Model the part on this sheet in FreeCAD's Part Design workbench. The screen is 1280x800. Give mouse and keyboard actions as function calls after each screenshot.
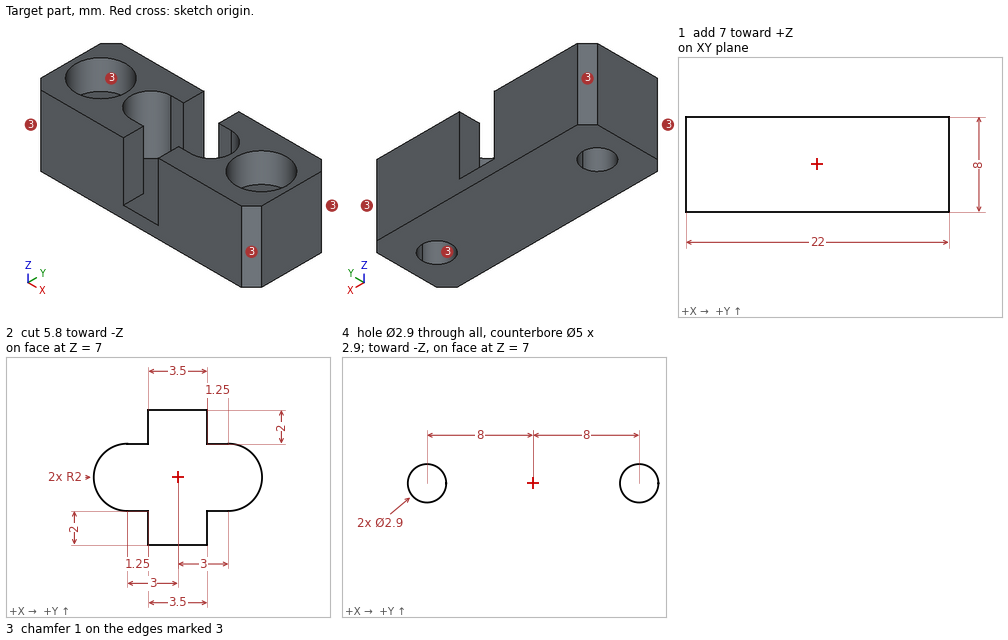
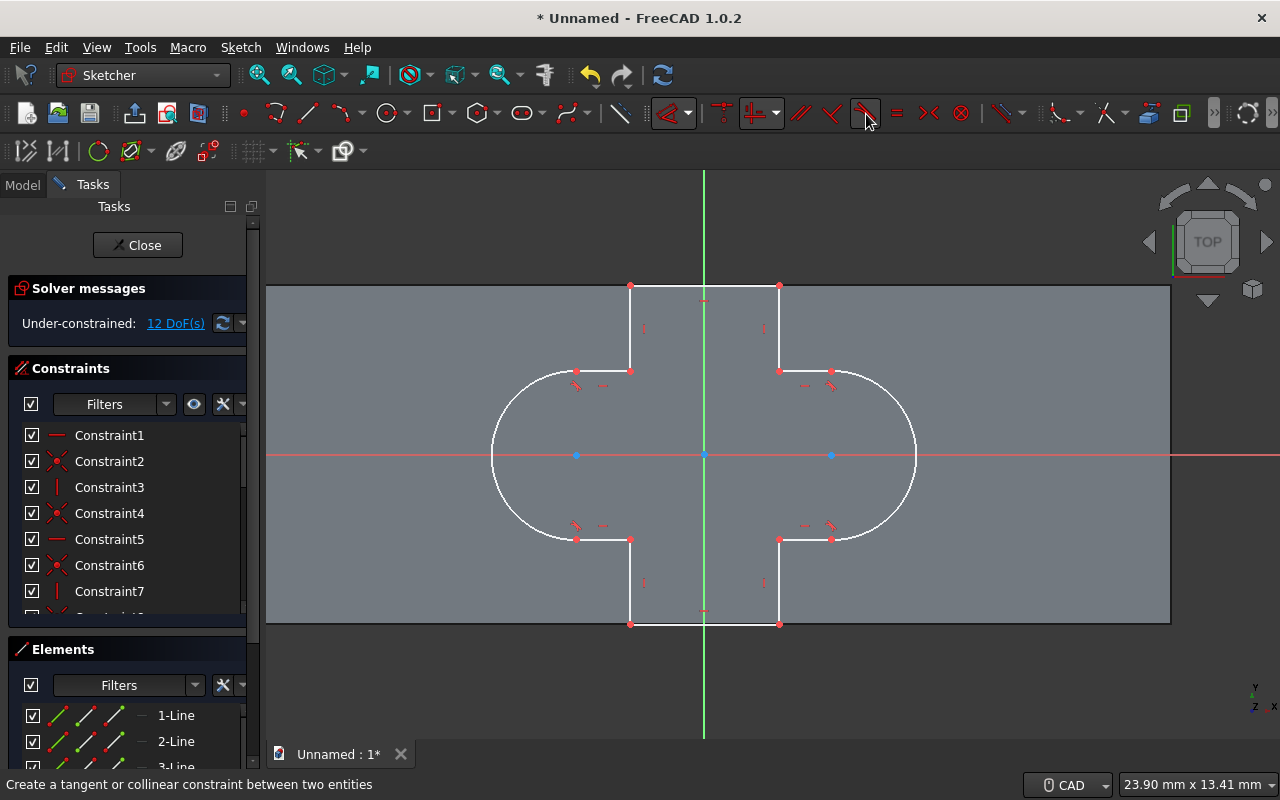
click(900, 505)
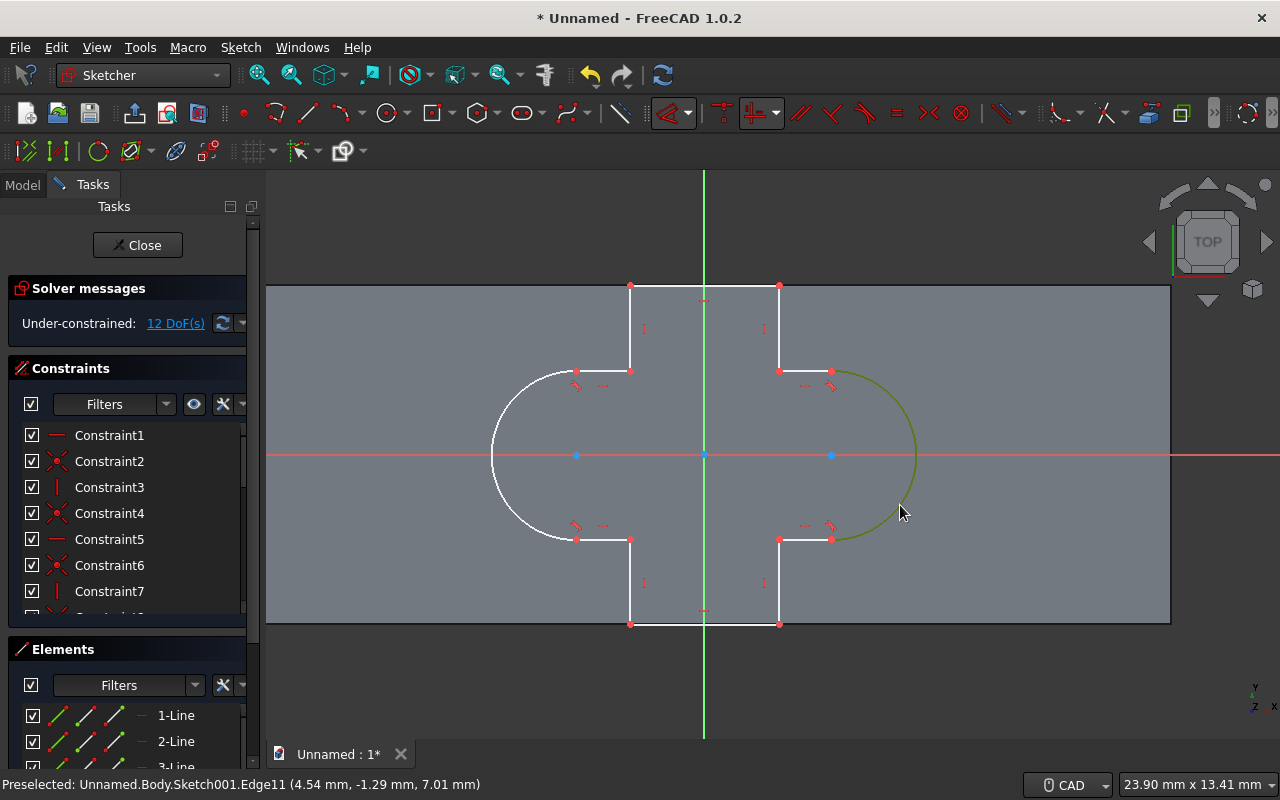
click(508, 406)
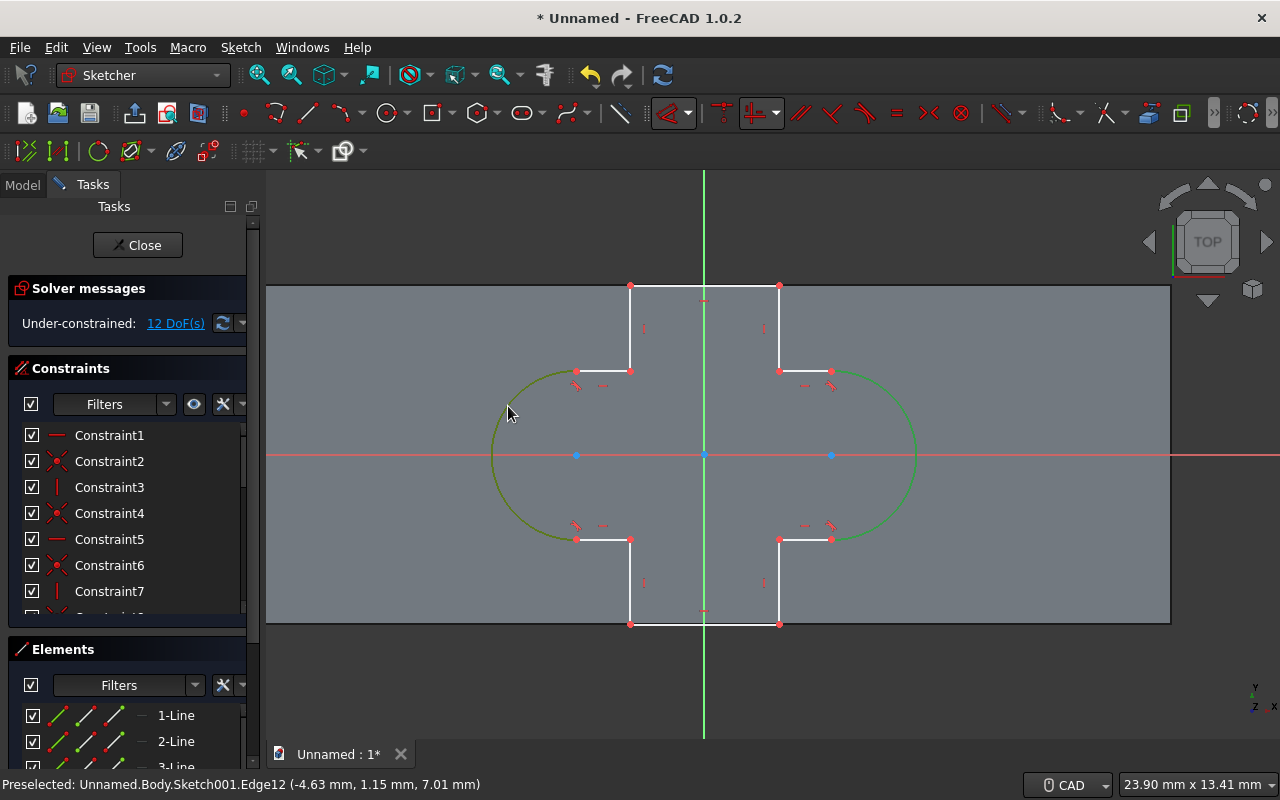
click(898, 114)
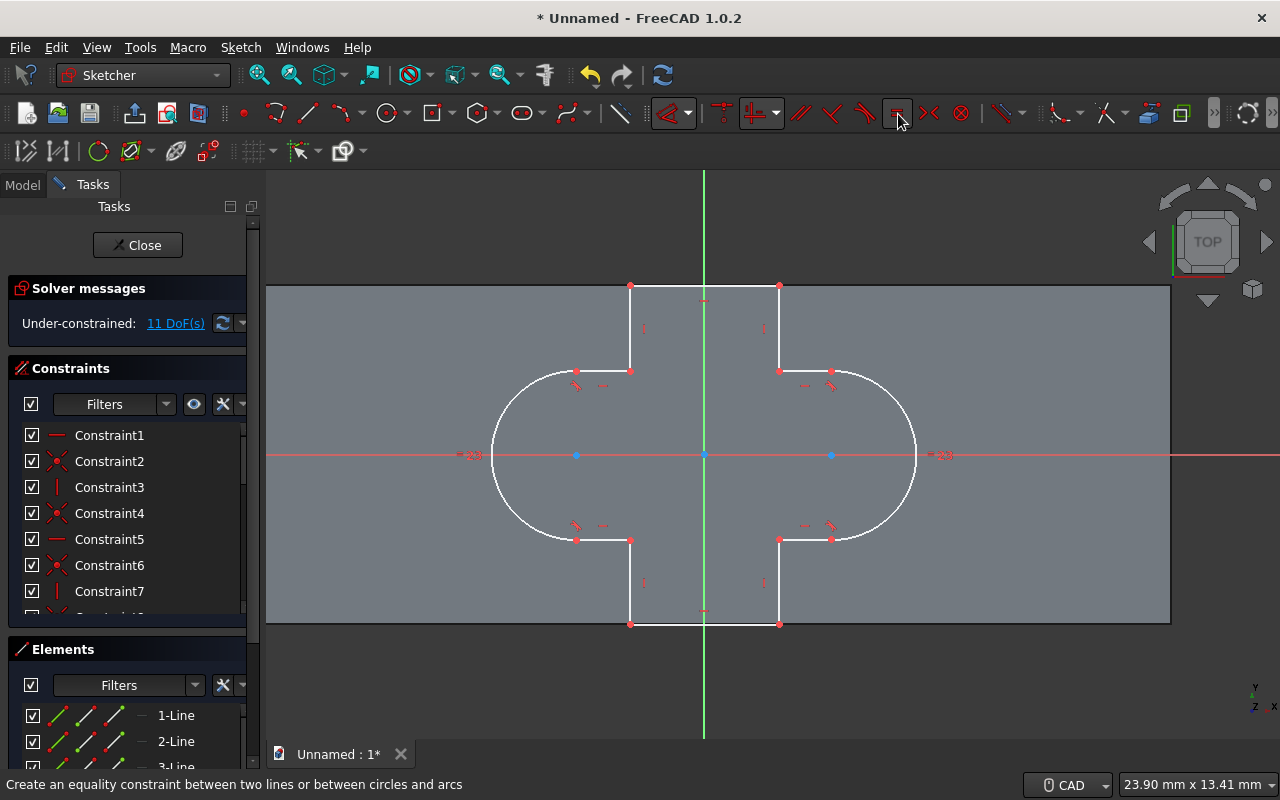
click(832, 456)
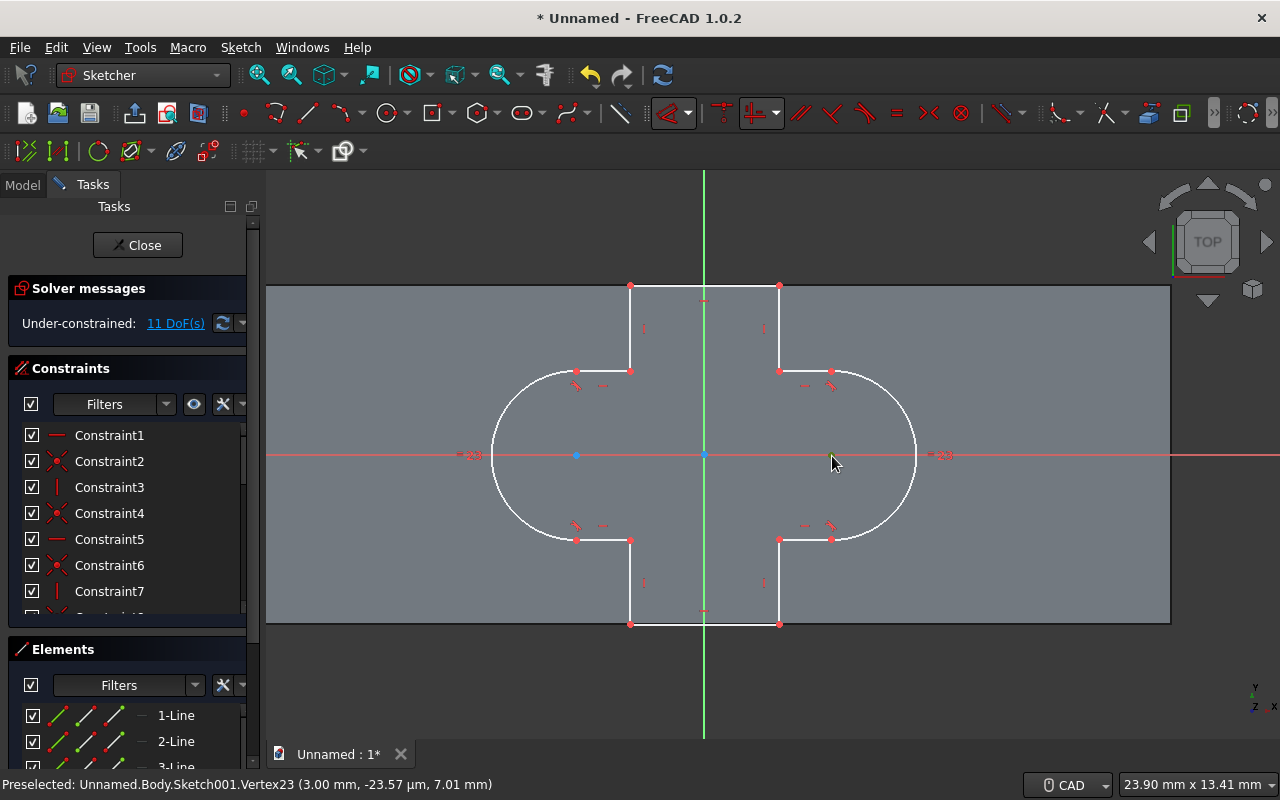
click(353, 454)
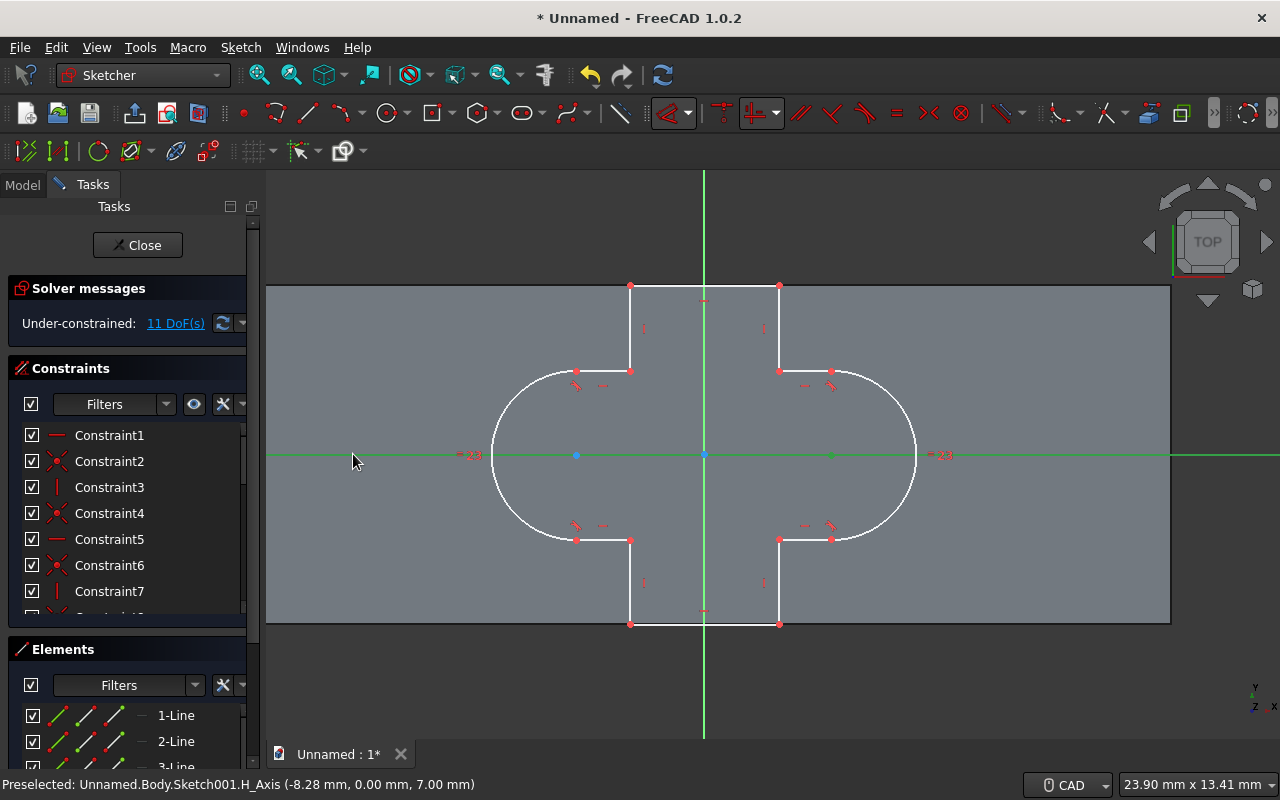
click(722, 114)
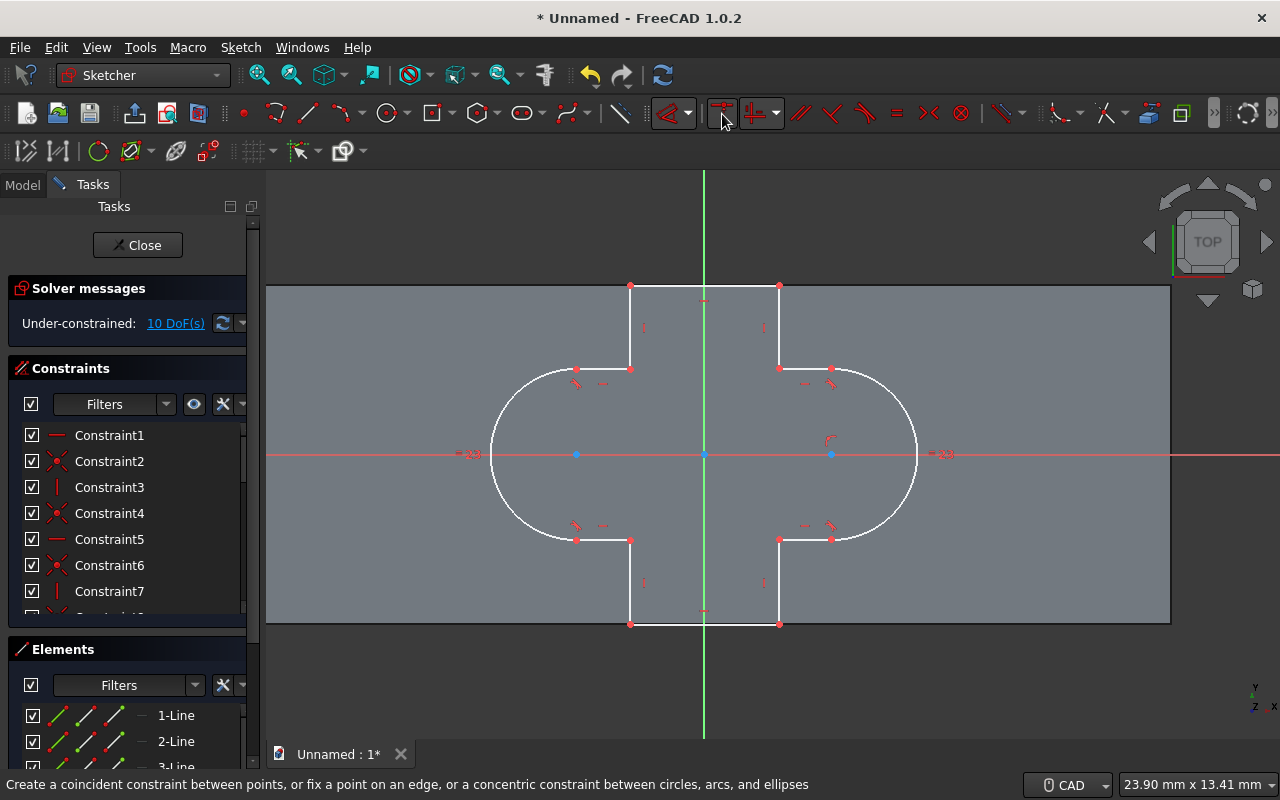
click(576, 455)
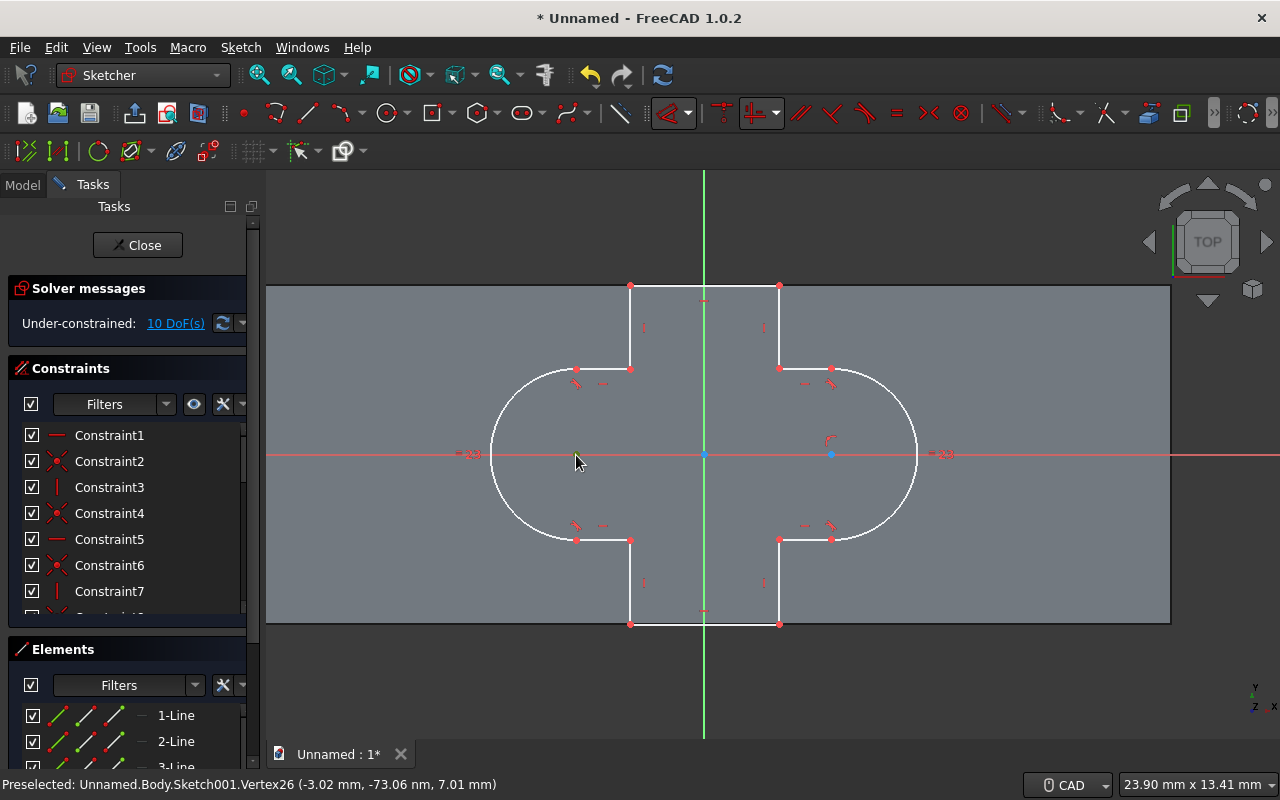
click(353, 454)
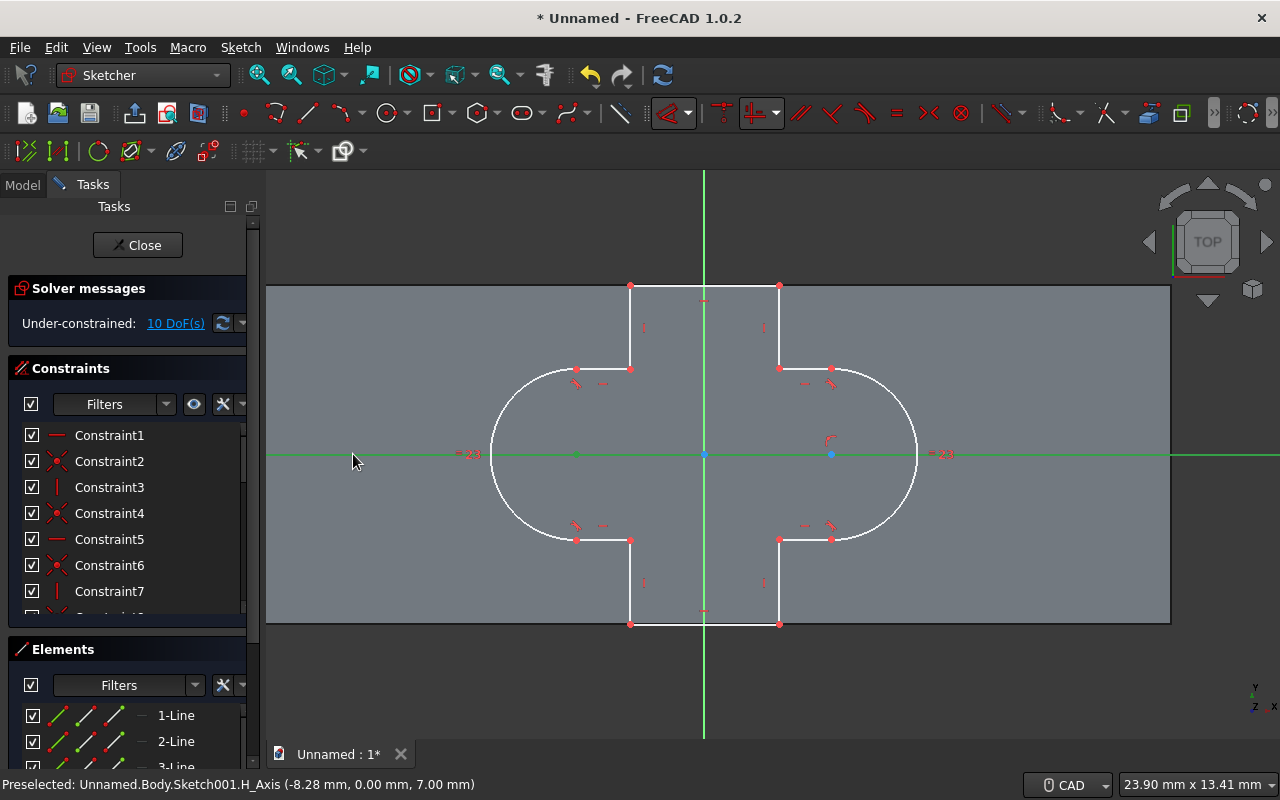
click(722, 114)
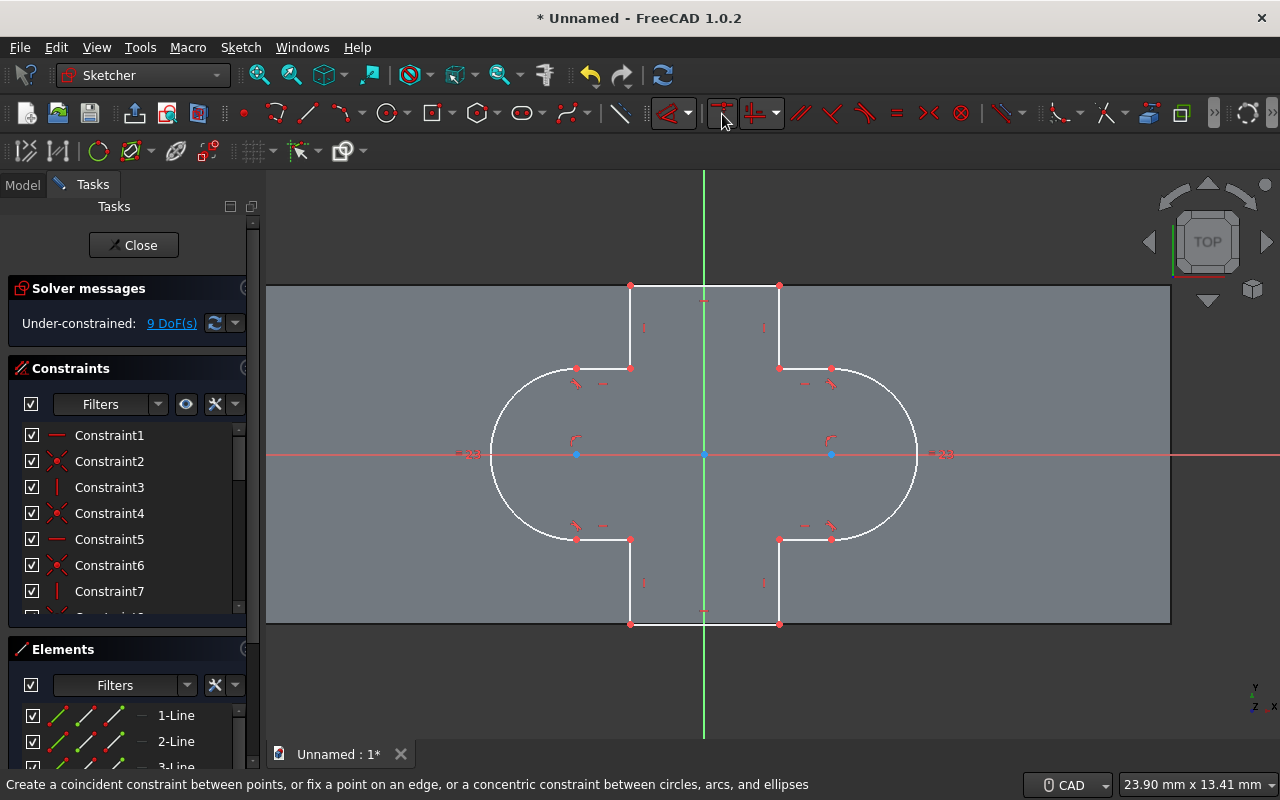
click(901, 505)